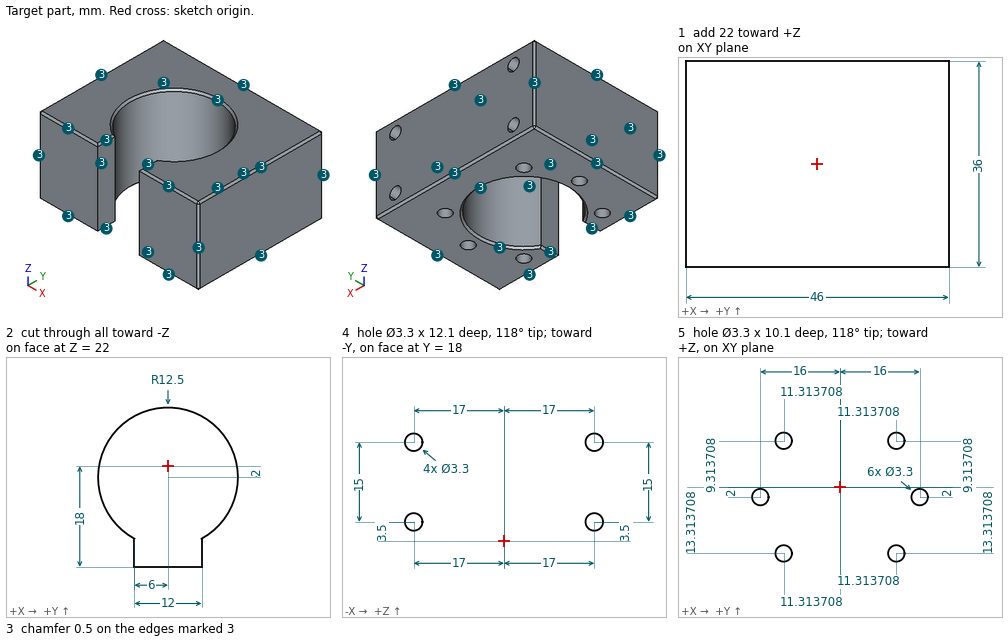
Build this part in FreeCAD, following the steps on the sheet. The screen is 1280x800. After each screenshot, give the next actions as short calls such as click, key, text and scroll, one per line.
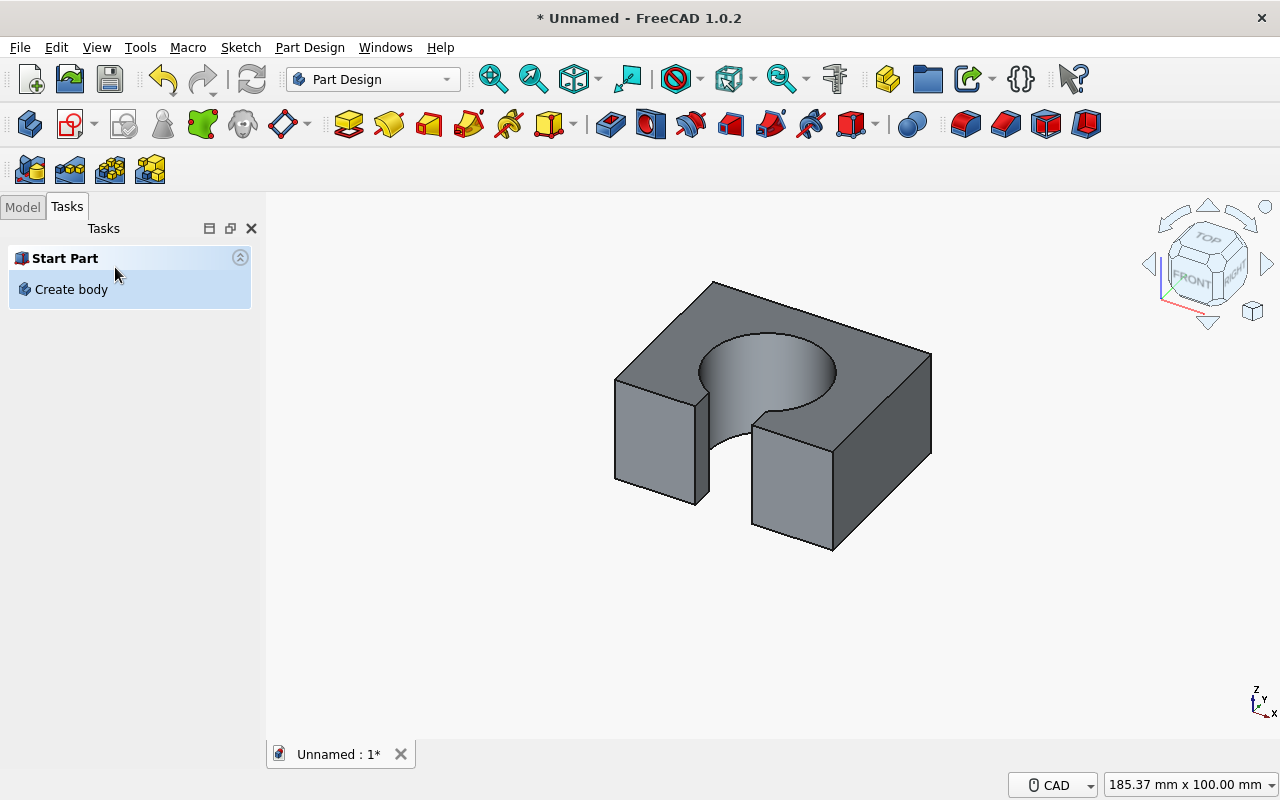
click(863, 359)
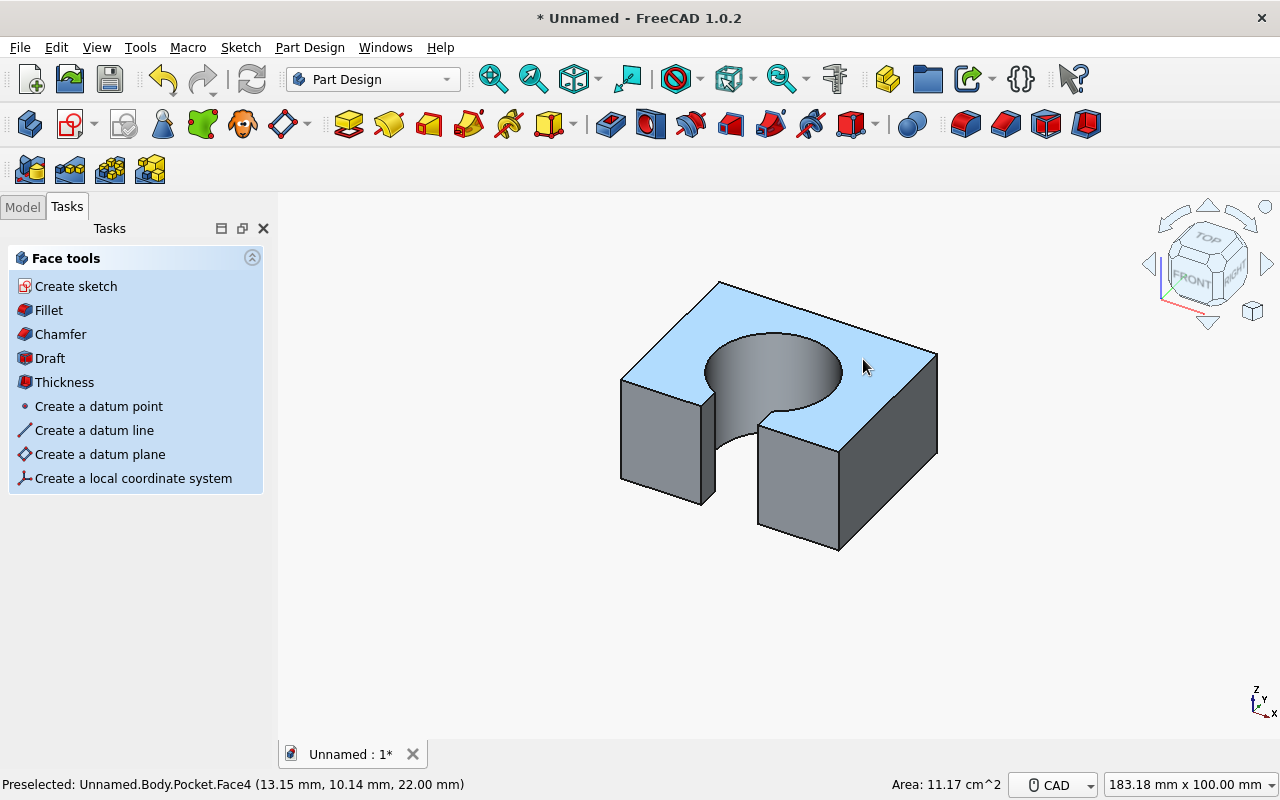
click(839, 500, ctrl)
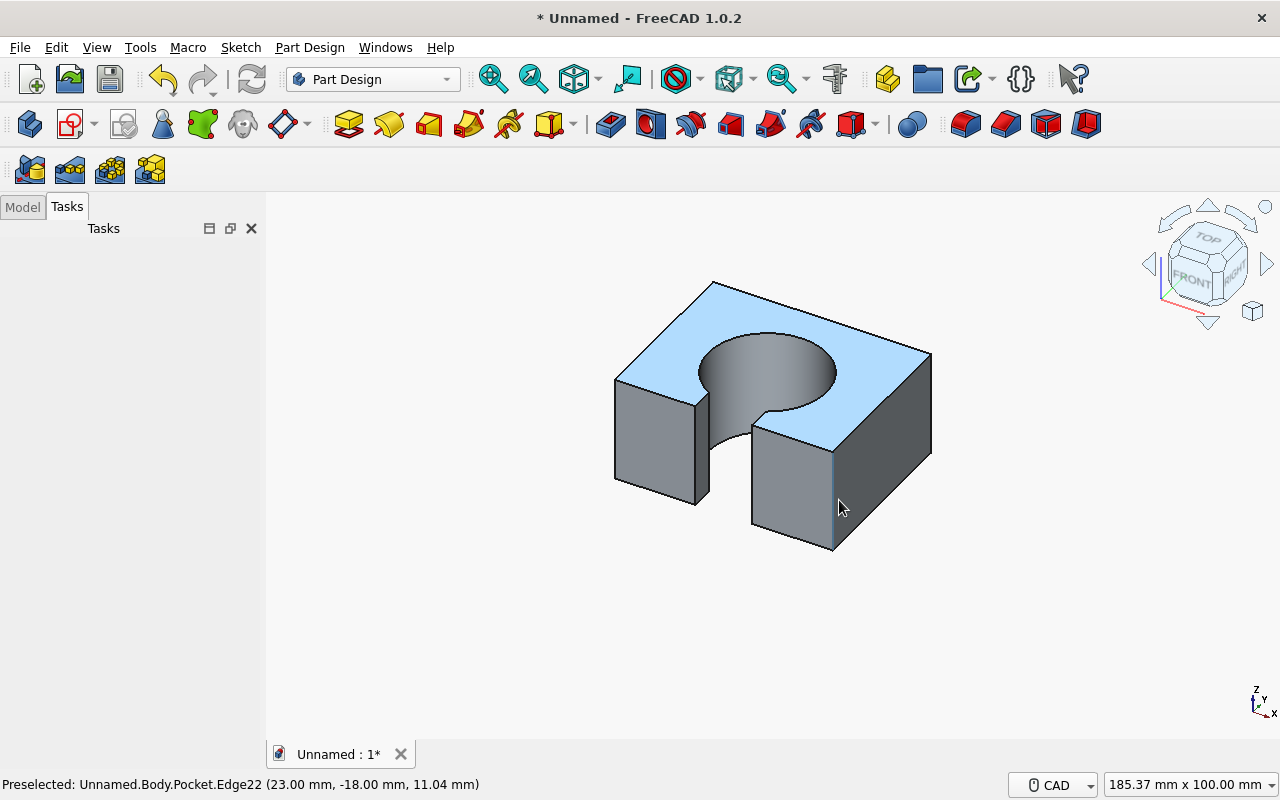
key(0)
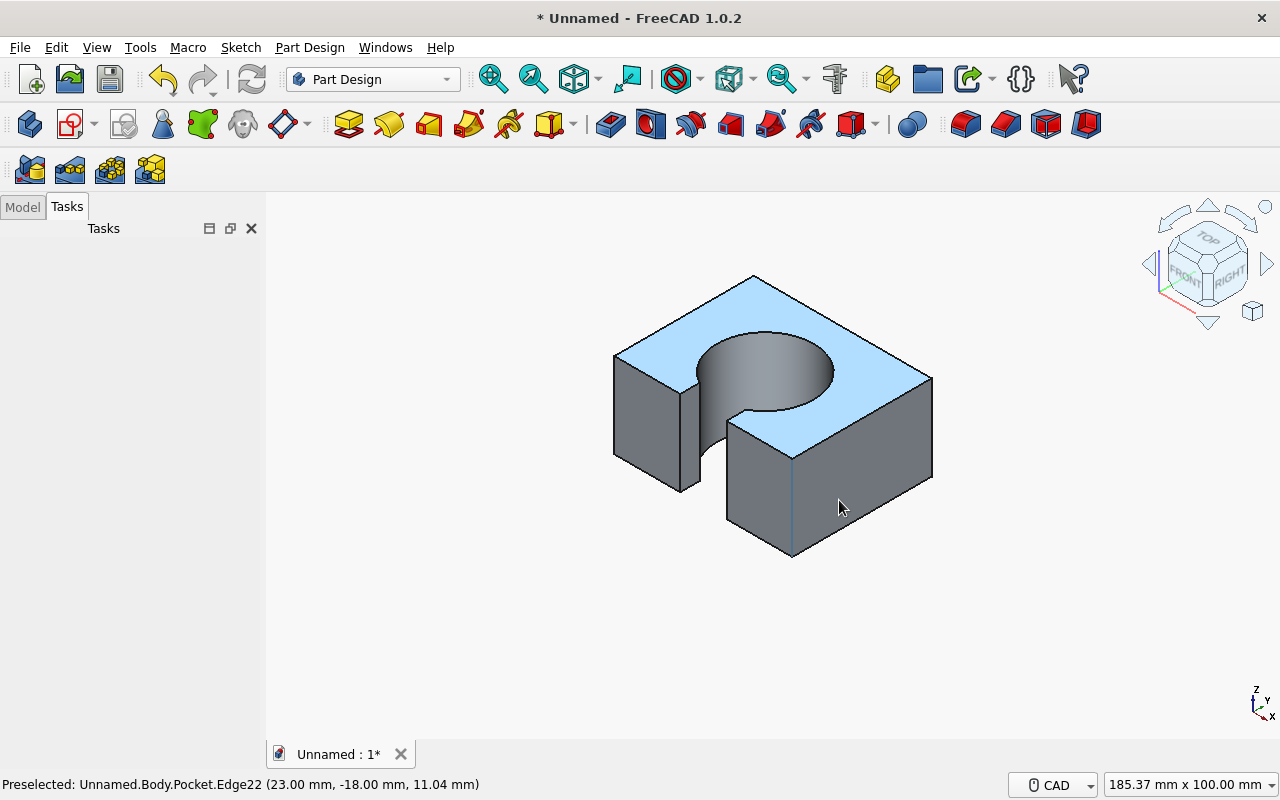
key(2)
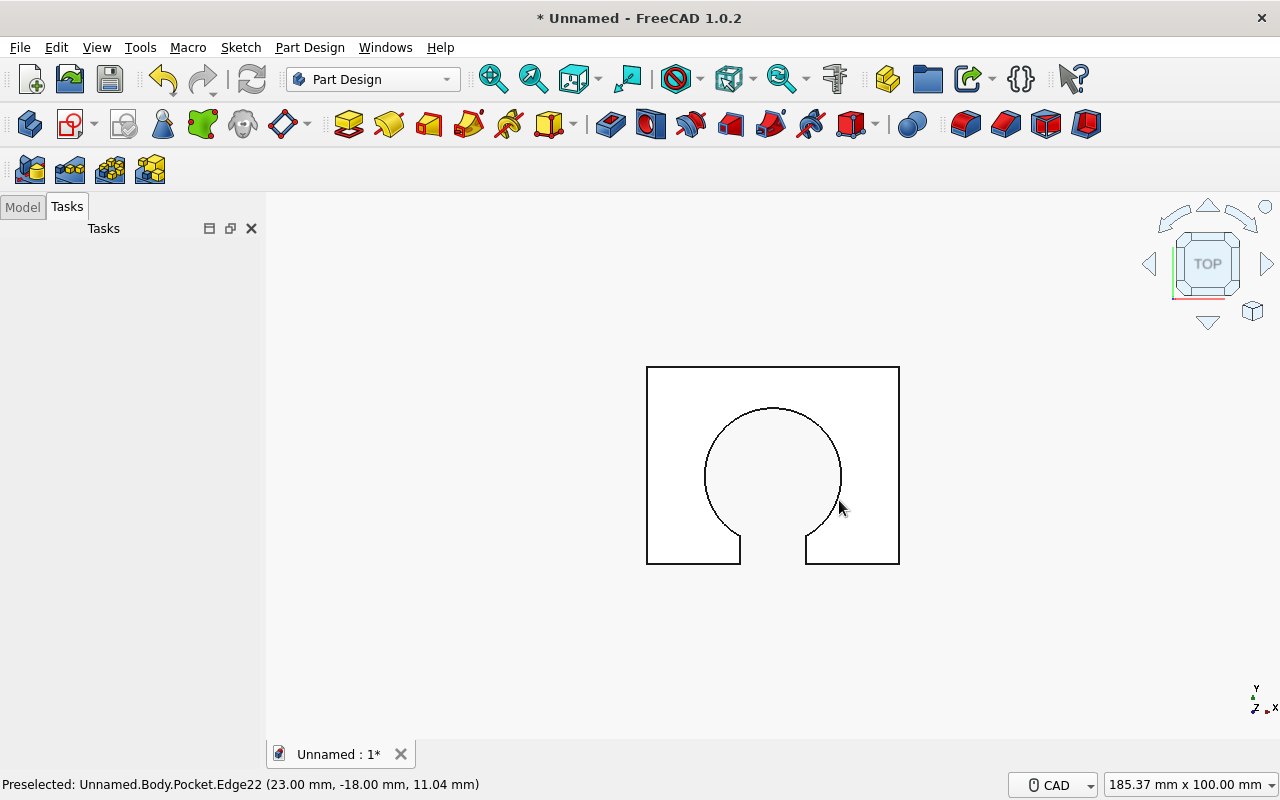
click(494, 80)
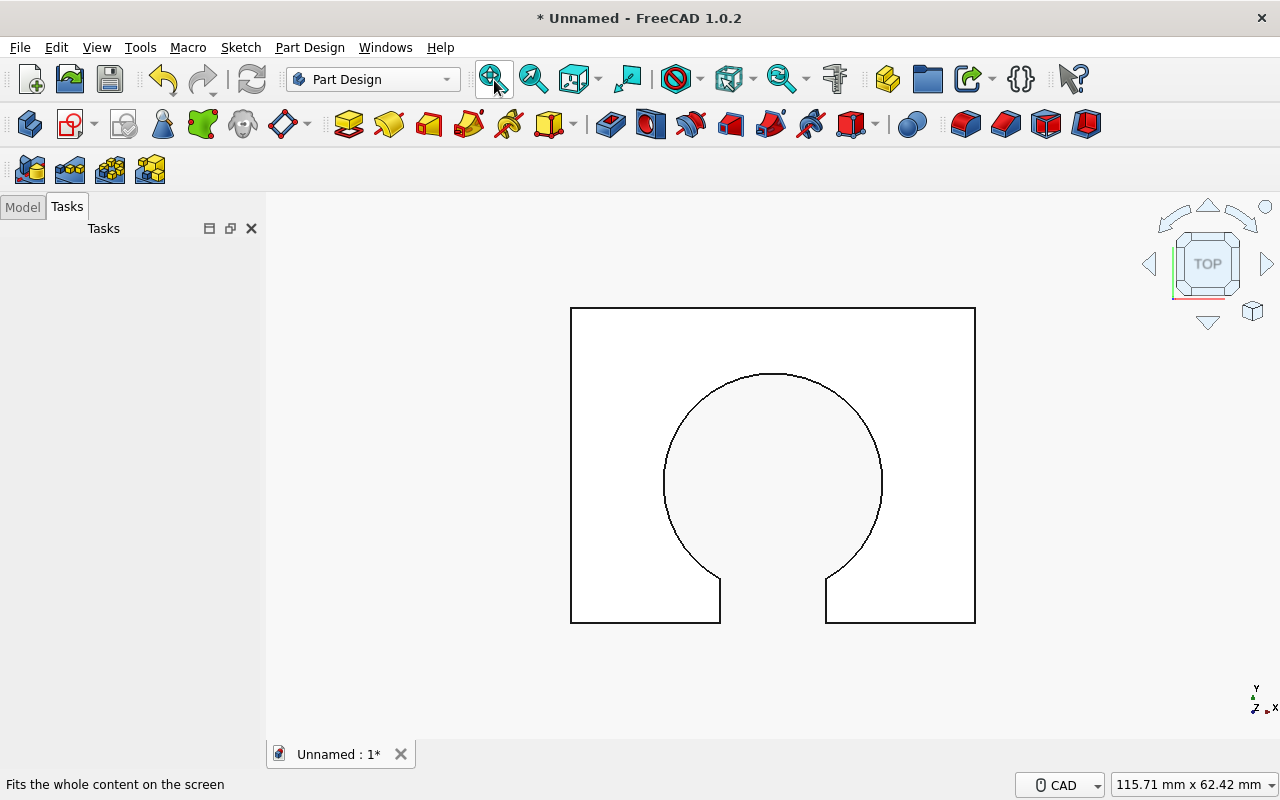
key(1)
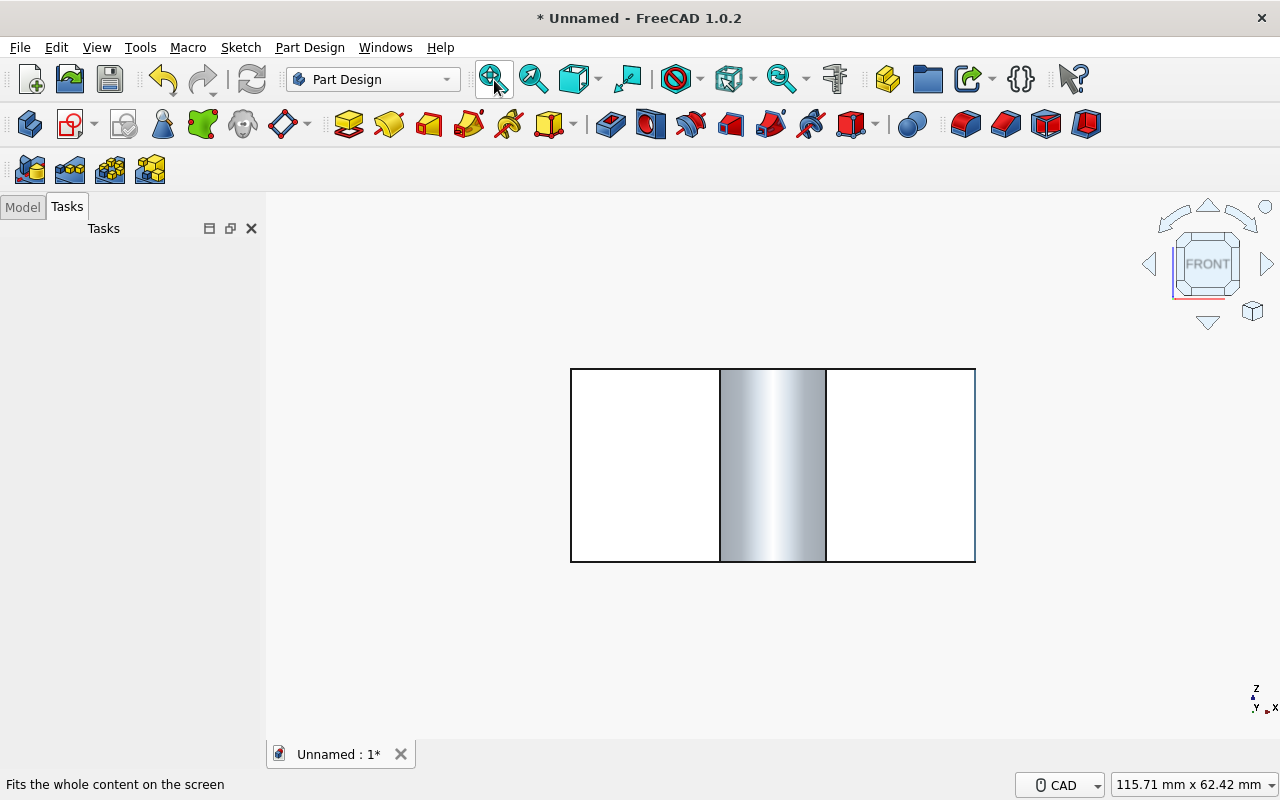
key(v)
key(f)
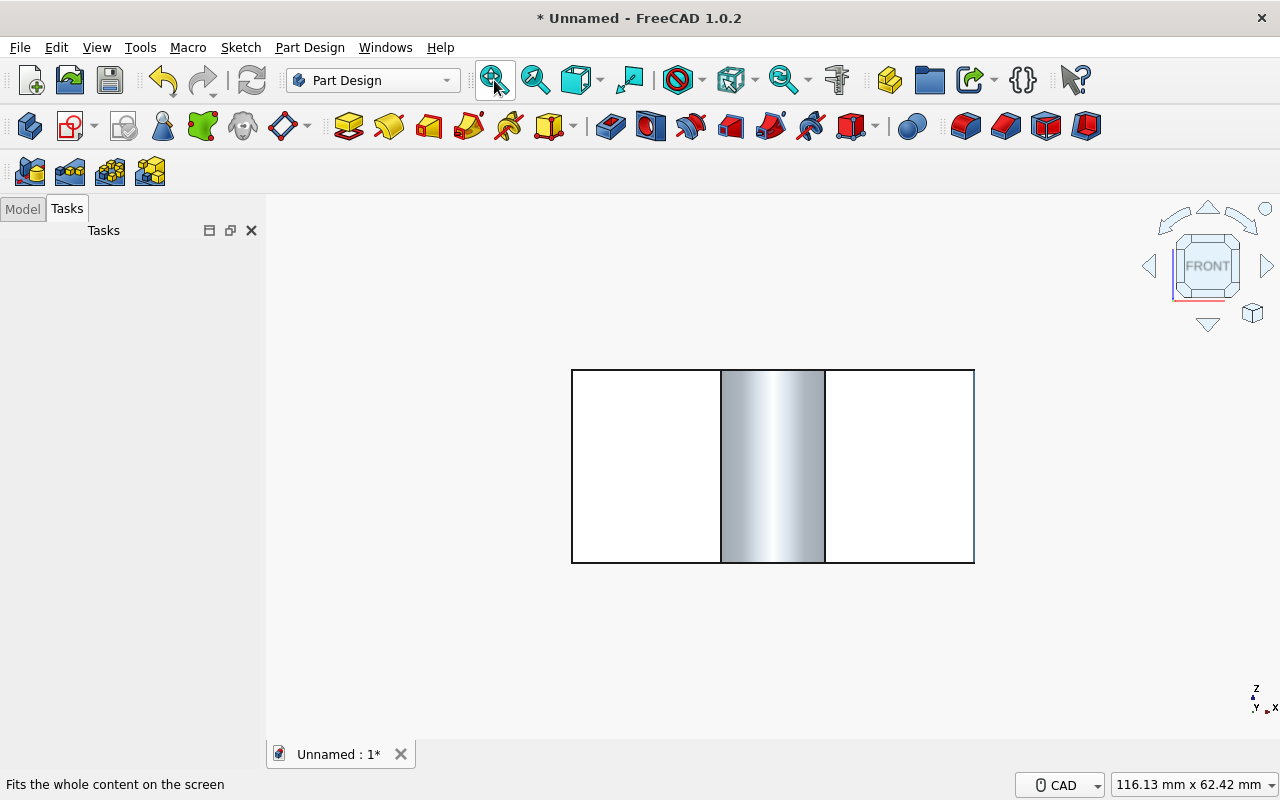
click(572, 466, ctrl)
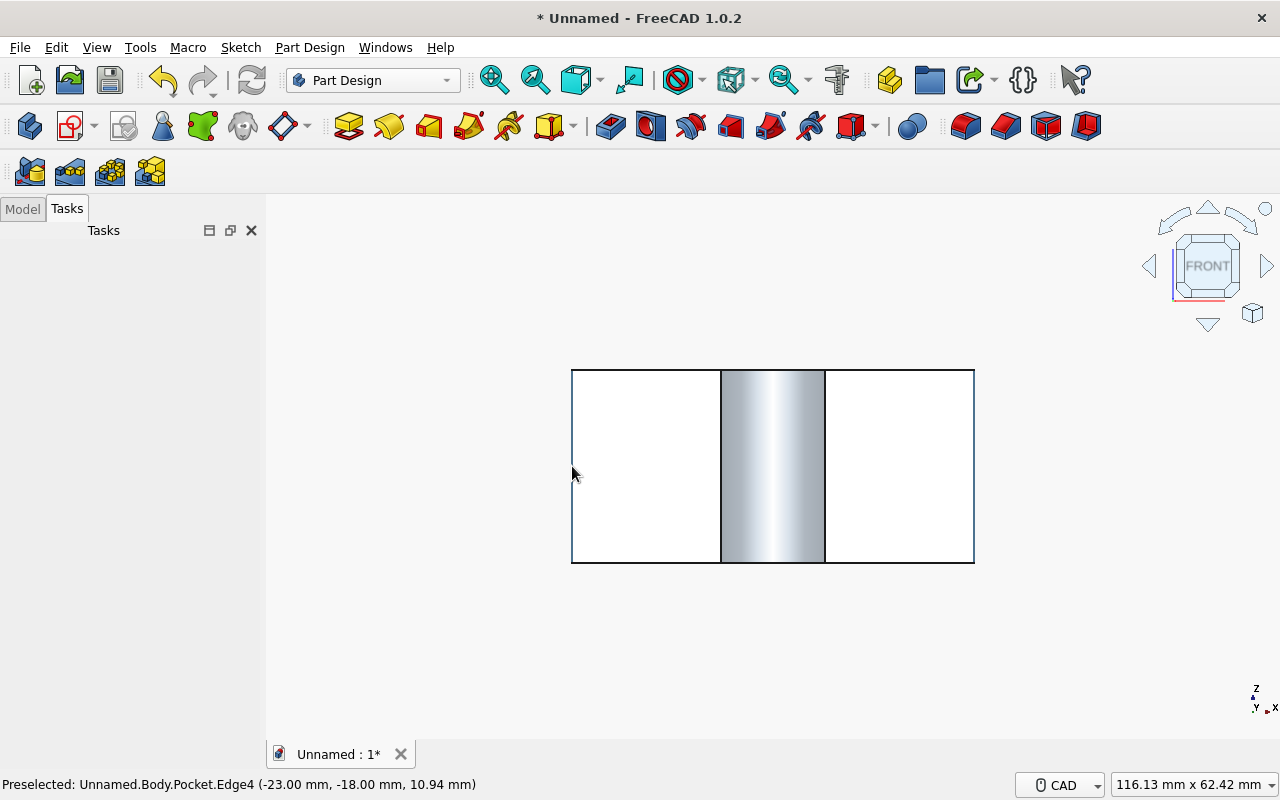
key(3)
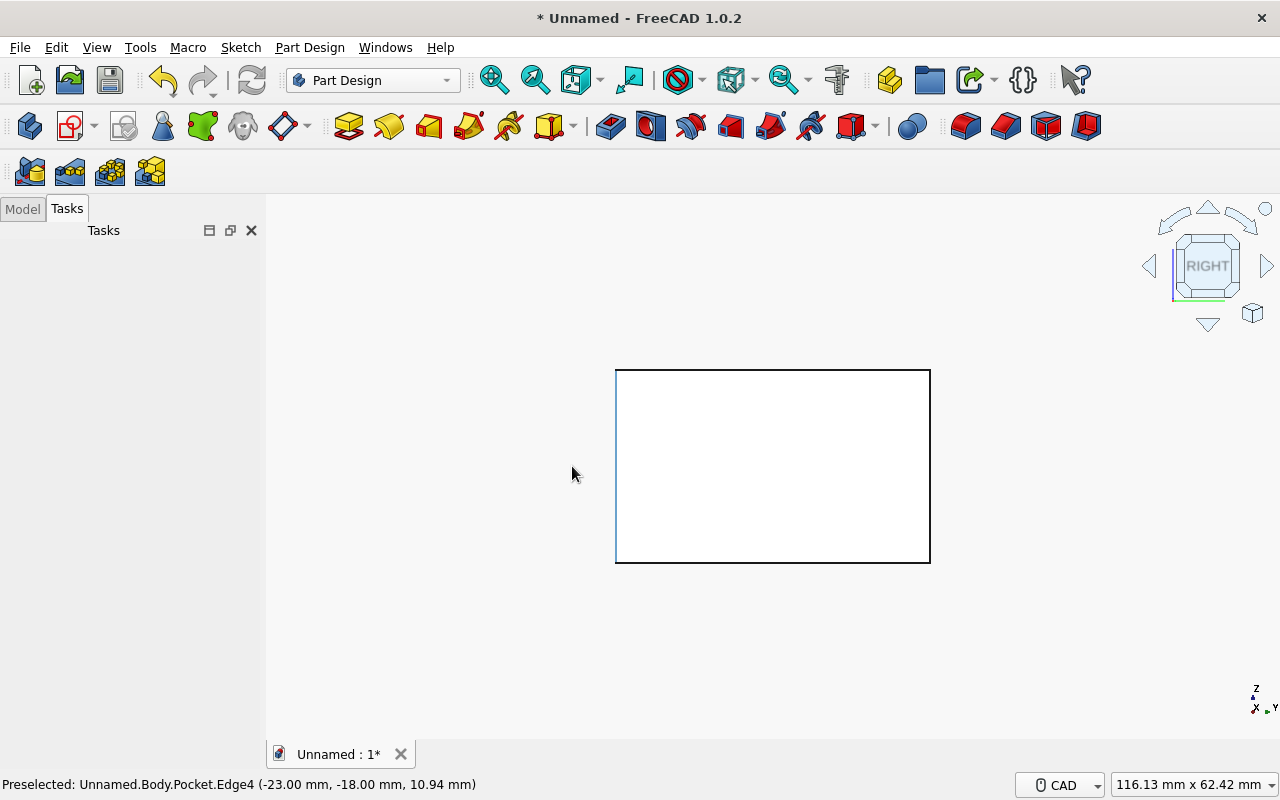
click(496, 80)